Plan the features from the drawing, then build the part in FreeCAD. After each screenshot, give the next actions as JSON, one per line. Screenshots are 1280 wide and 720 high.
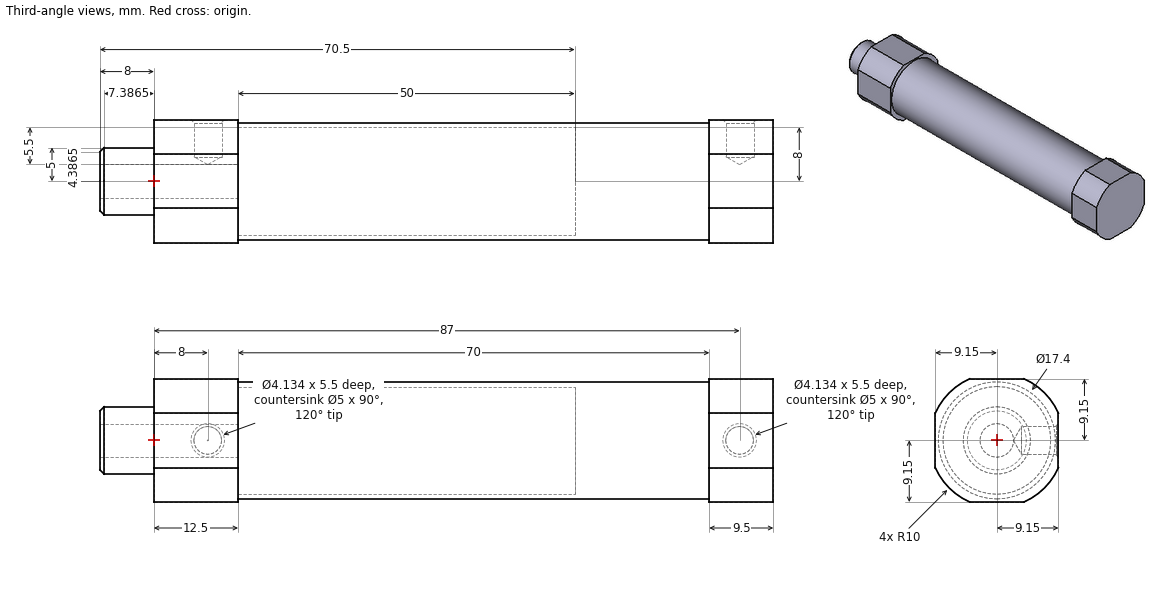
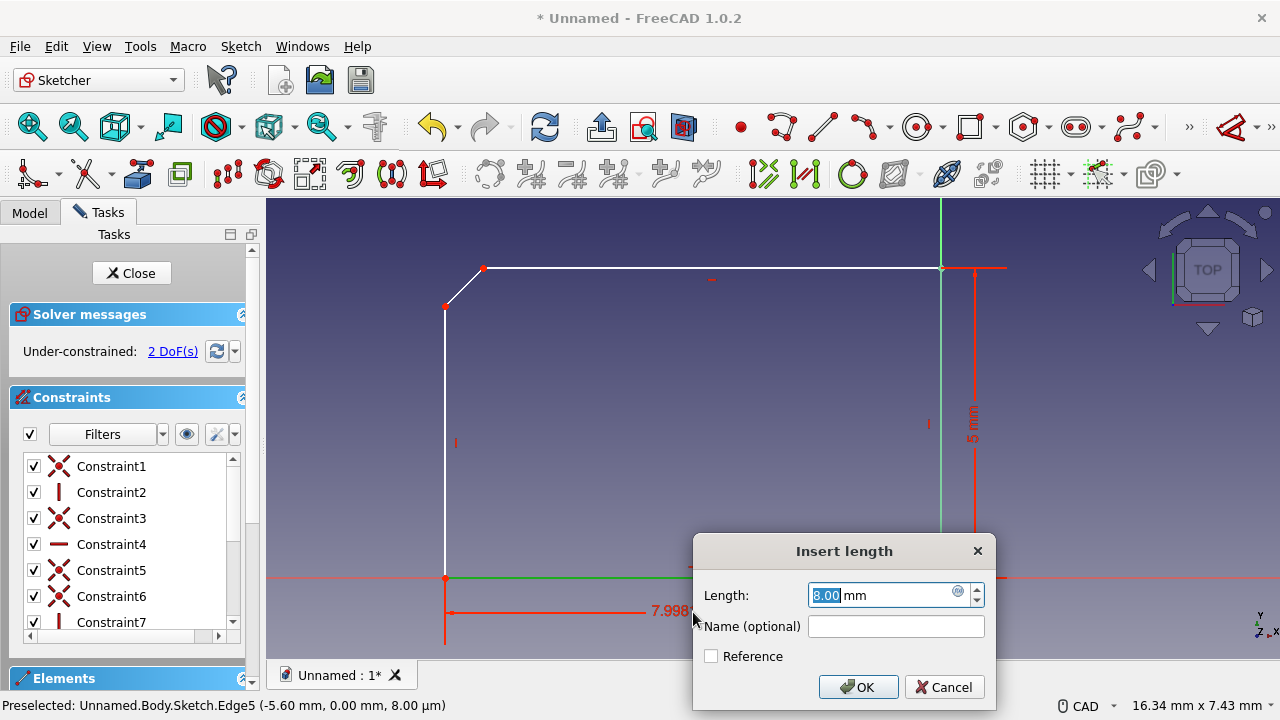
{"action": "type", "text": "8"}
{"action": "key", "text": "Return"}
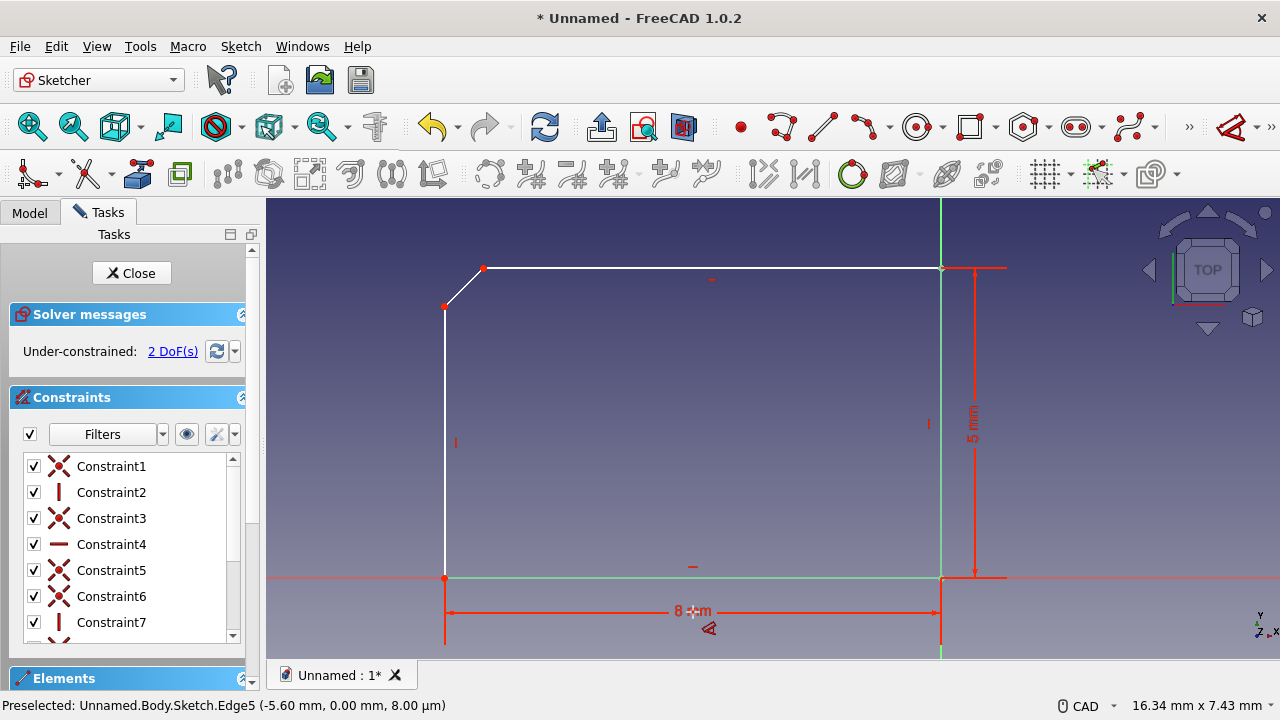
{"action": "left_click", "coordinate": [804, 268]}
{"action": "left_click", "coordinate": [712, 234]}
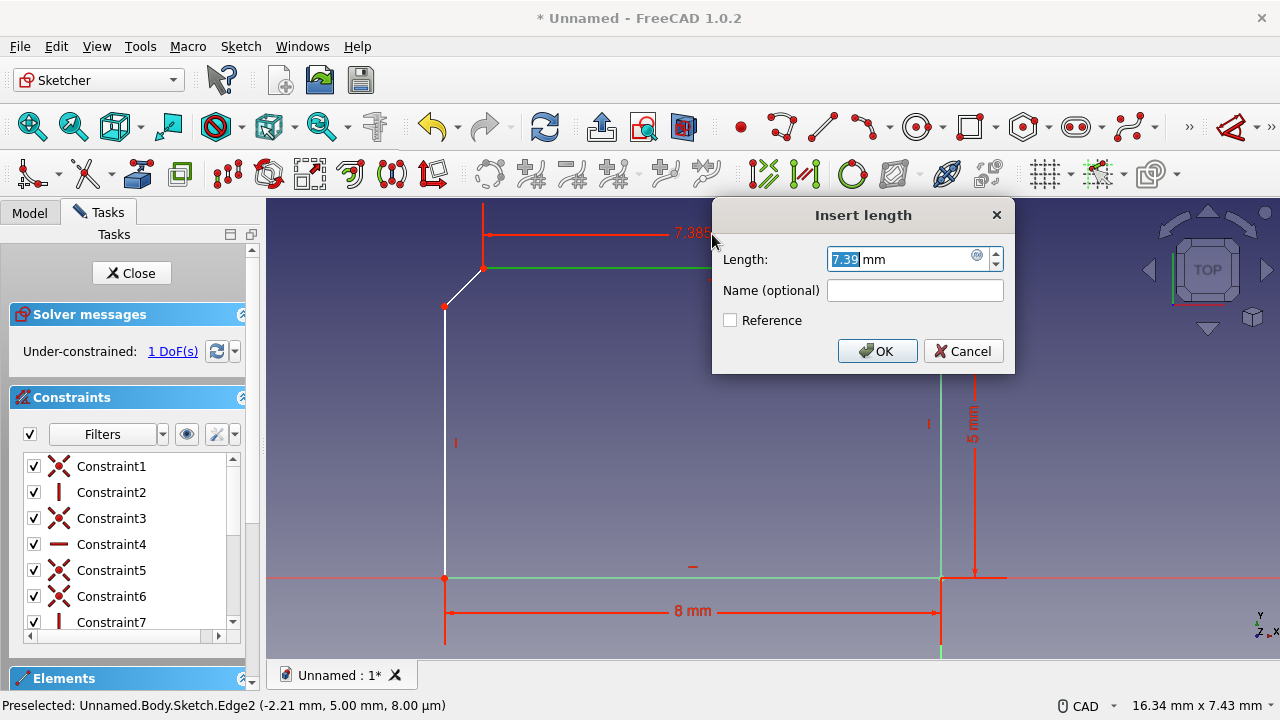
{"action": "type", "text": "7.3865"}
{"action": "key", "text": "Return"}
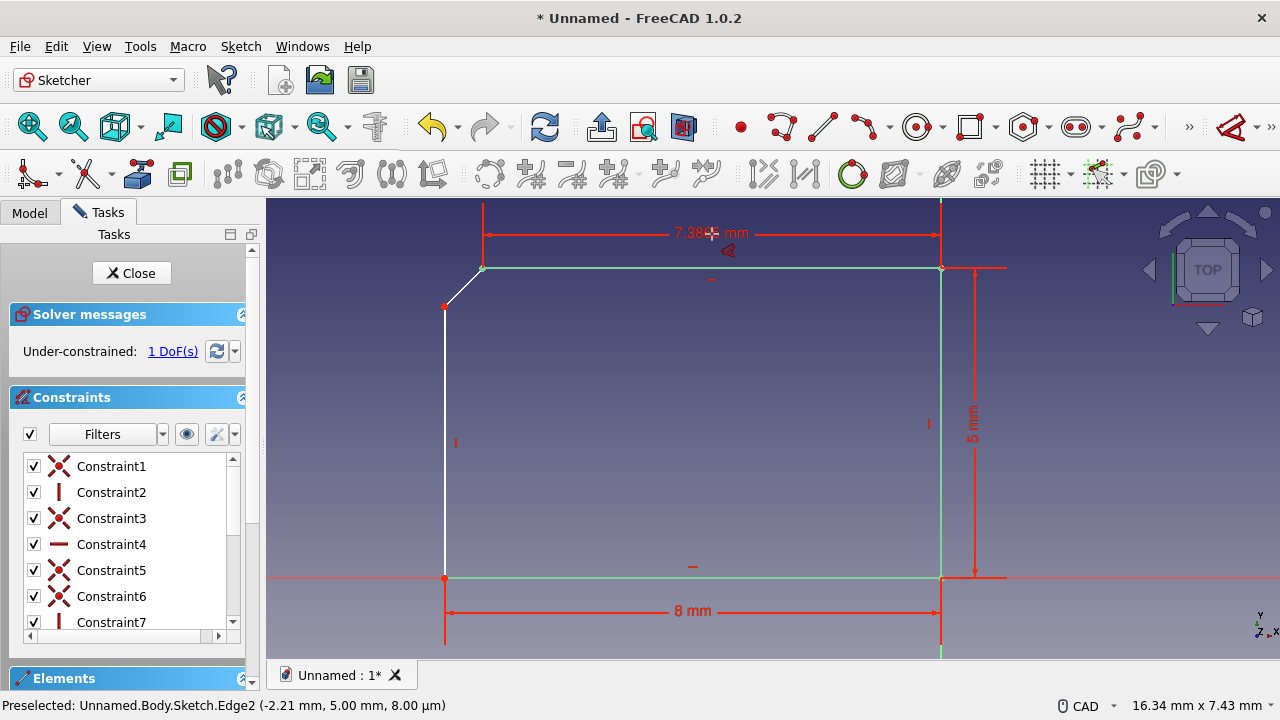
{"action": "left_click", "coordinate": [445, 388]}
{"action": "left_click", "coordinate": [411, 443]}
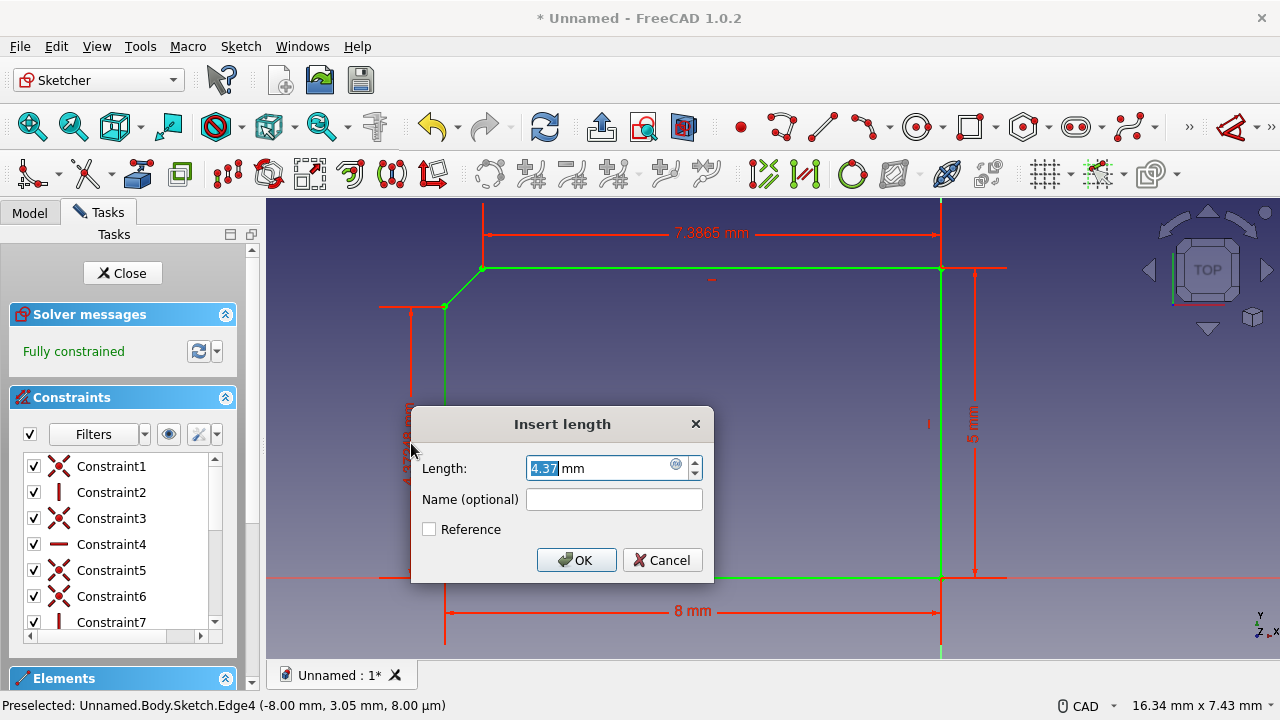
{"action": "type", "text": "4.3865"}
{"action": "key", "text": "Return"}
{"action": "key", "text": "Escape"}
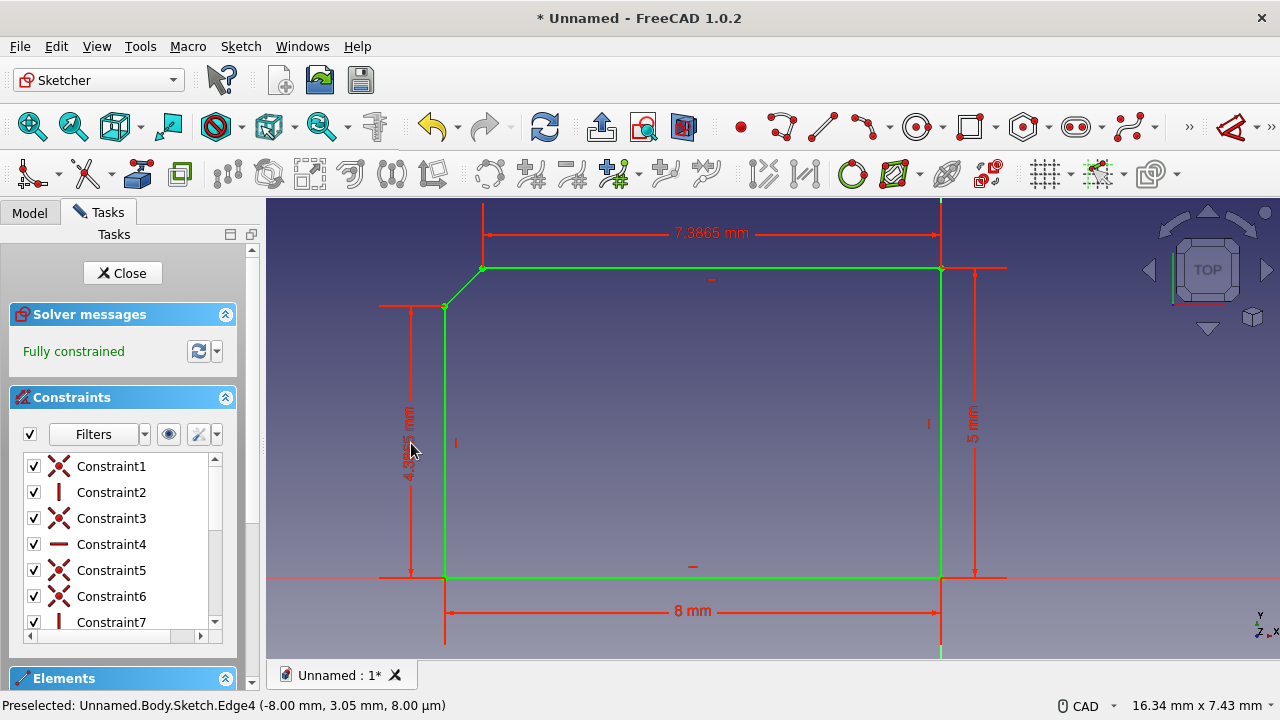
{"action": "left_click", "coordinate": [123, 273]}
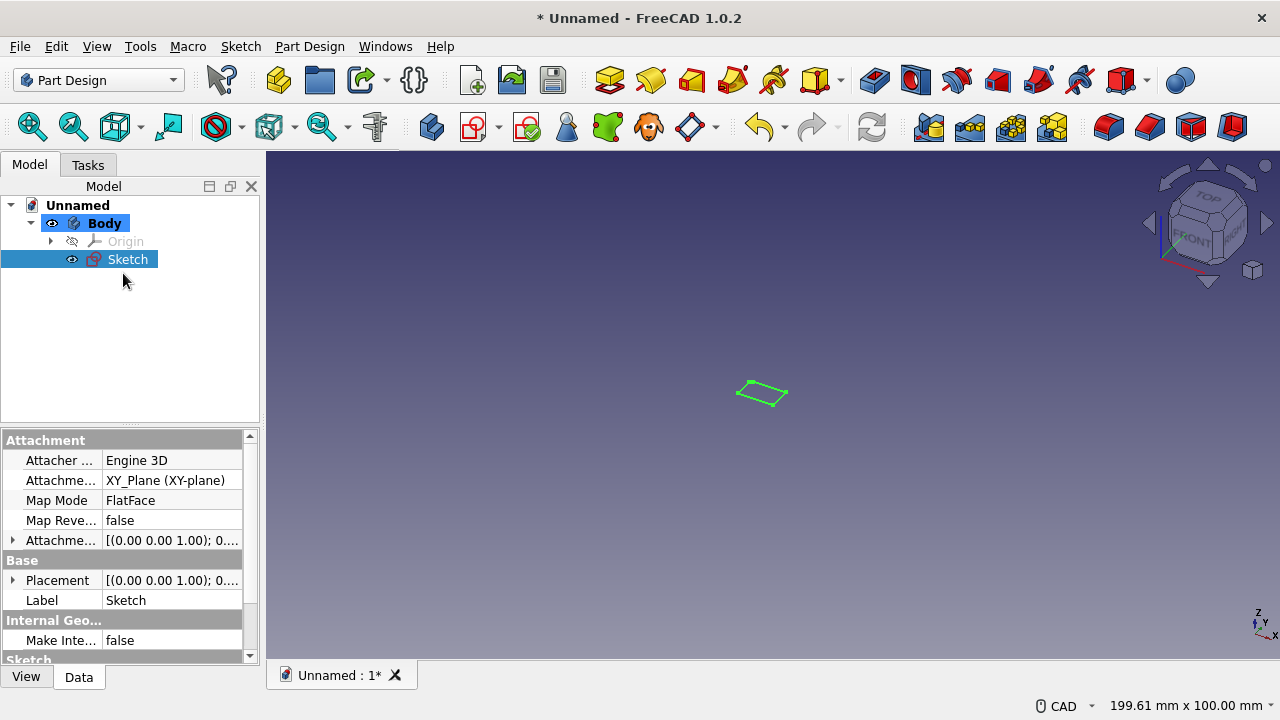
{"action": "left_click", "coordinate": [651, 80]}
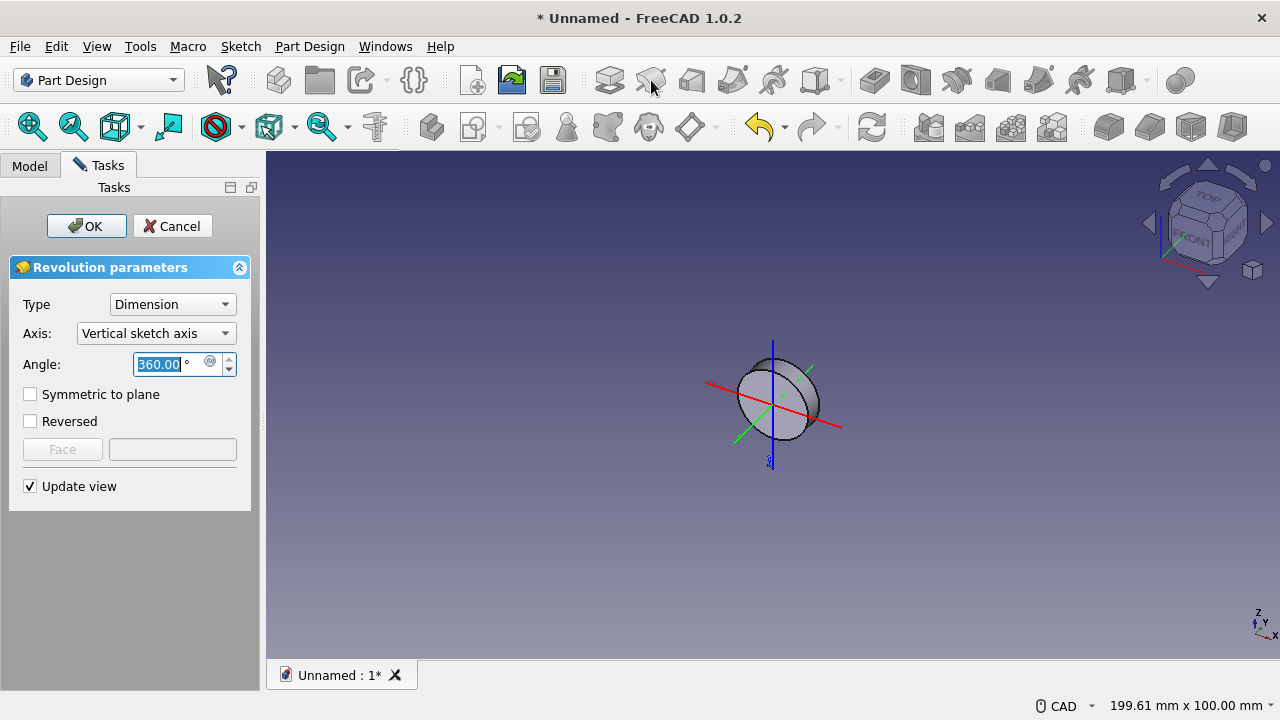
{"action": "left_click", "coordinate": [157, 334]}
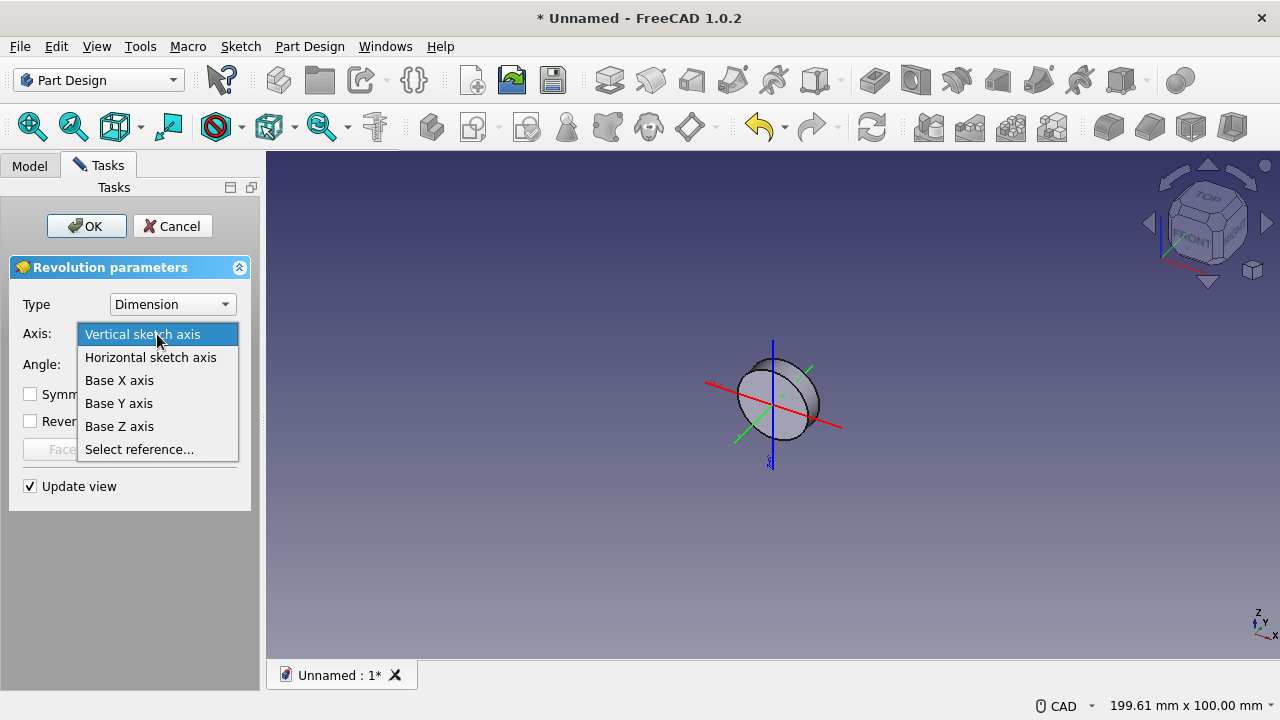
{"action": "left_click", "coordinate": [156, 358]}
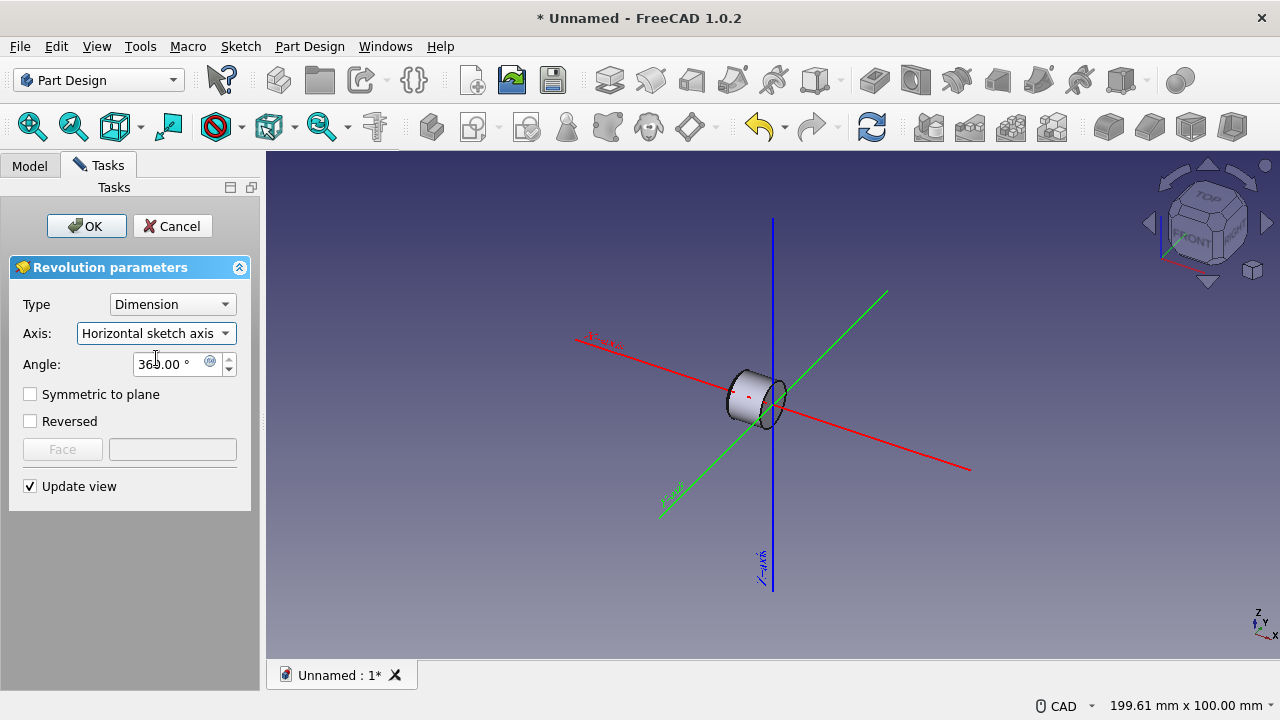
{"action": "left_click", "coordinate": [87, 226]}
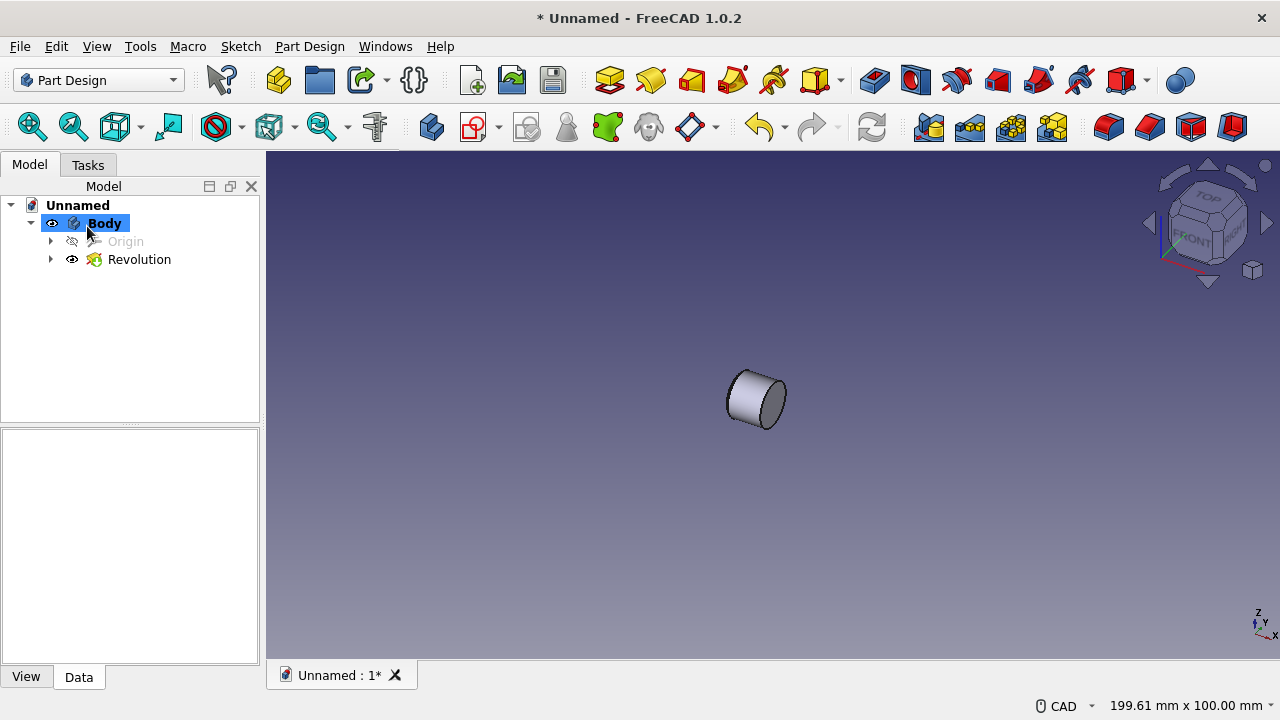
{"action": "left_click", "coordinate": [33, 128]}